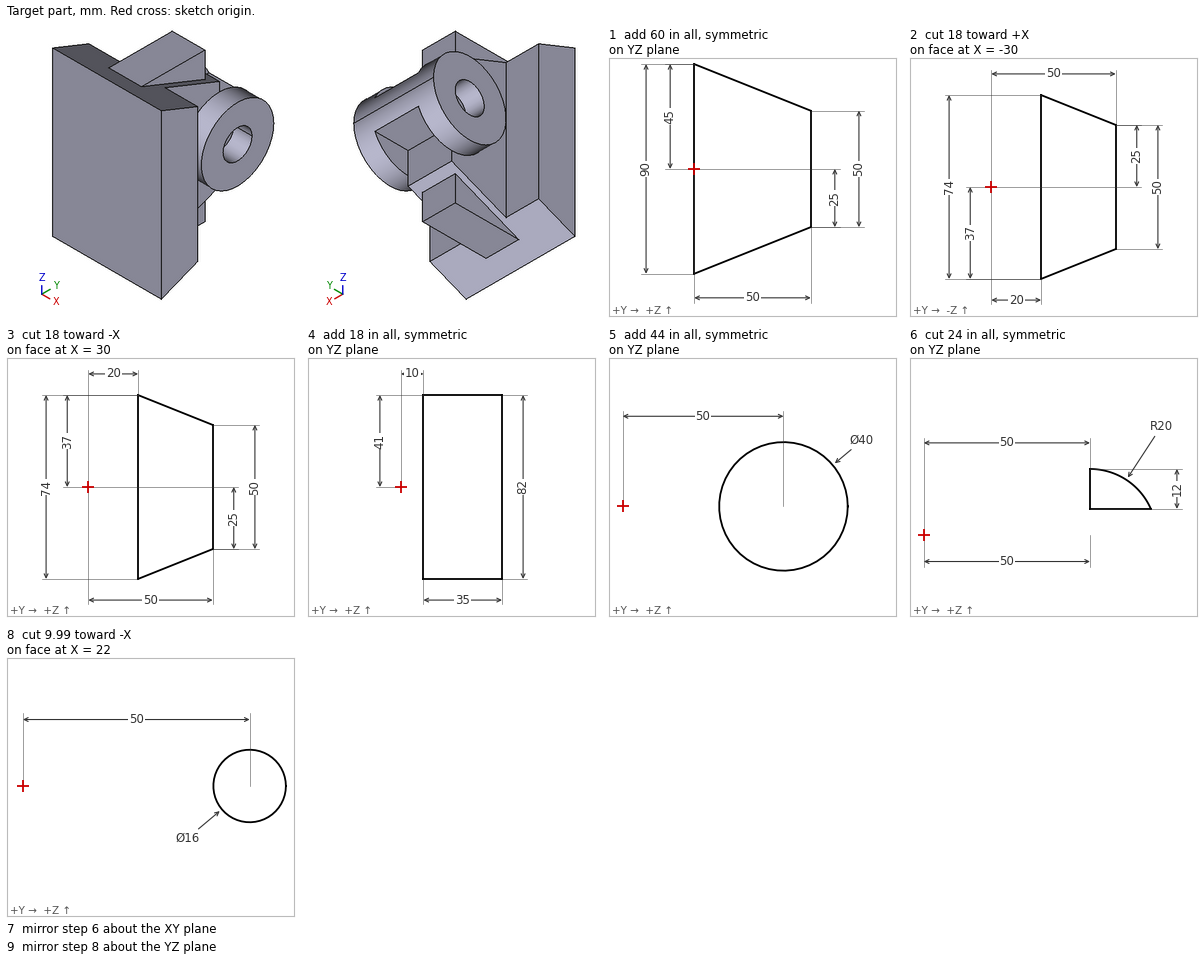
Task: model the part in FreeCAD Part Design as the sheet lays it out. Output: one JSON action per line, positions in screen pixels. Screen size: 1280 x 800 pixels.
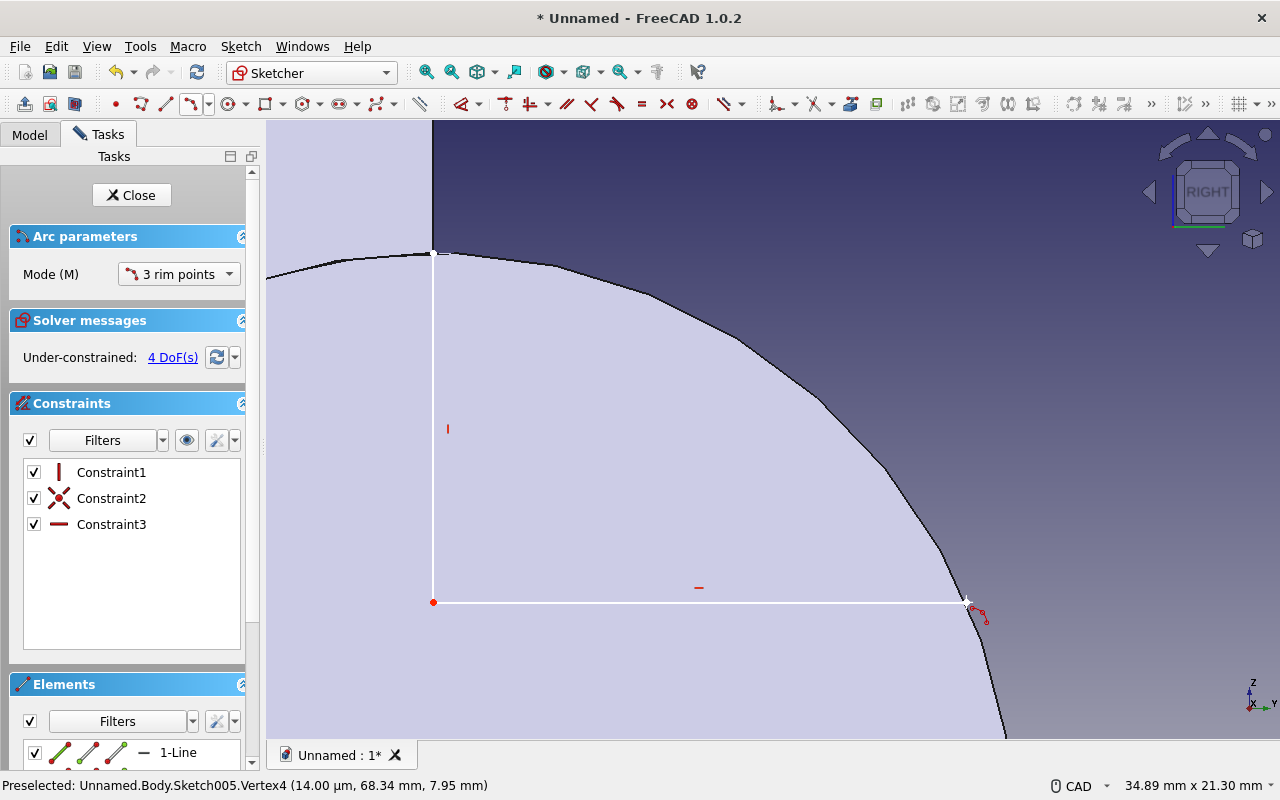
{"action": "left_click", "coordinate": [966, 603]}
{"action": "left_click", "coordinate": [433, 254]}
{"action": "left_click", "coordinate": [751, 348]}
{"action": "key", "text": "Escape"}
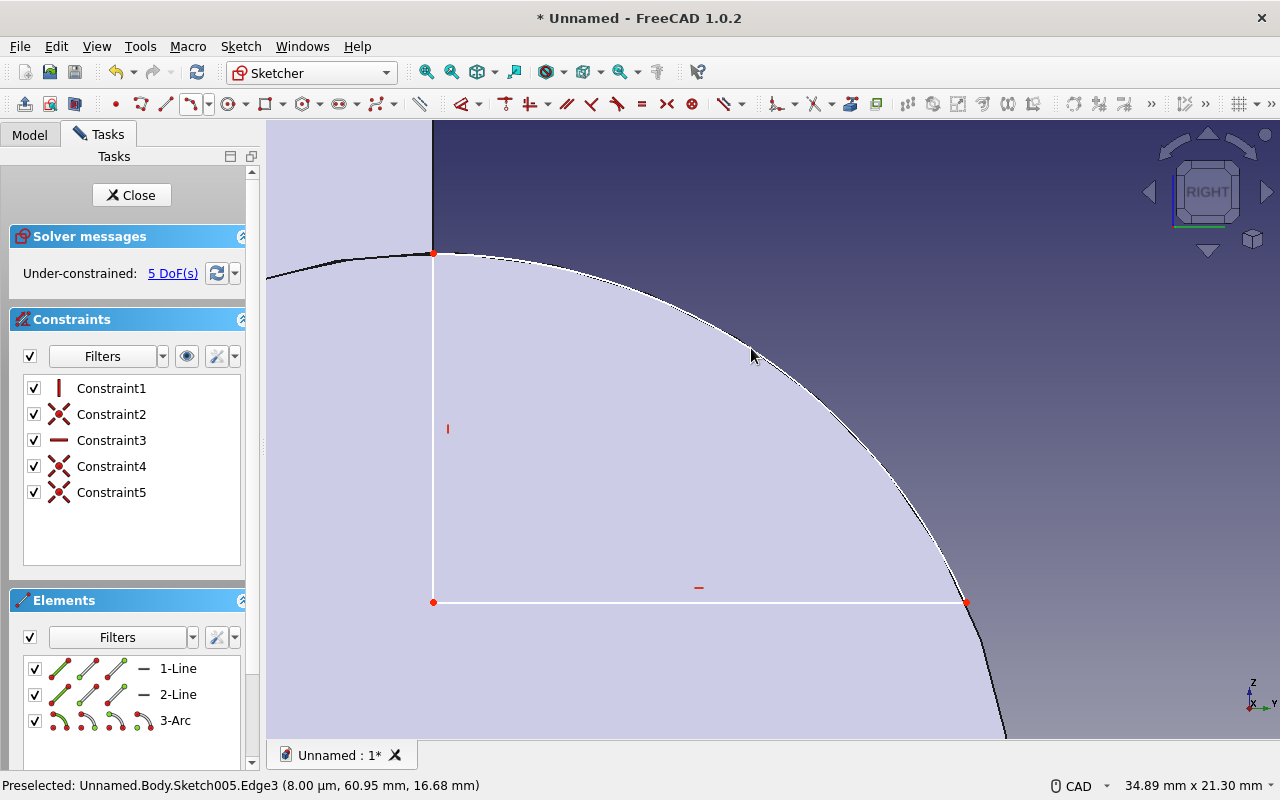
{"action": "scroll", "coordinate": [716, 195], "scroll_direction": "down", "scroll_amount": 2}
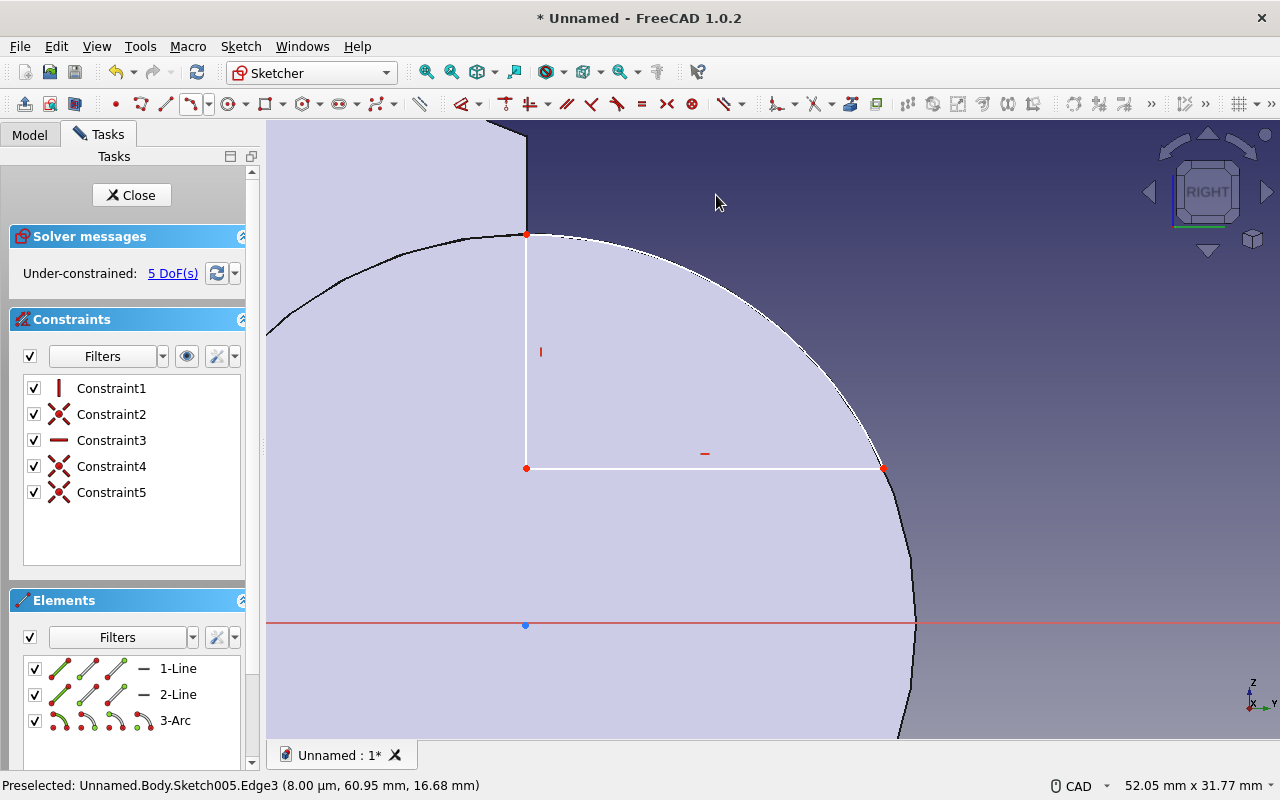
{"action": "left_click", "coordinate": [526, 625]}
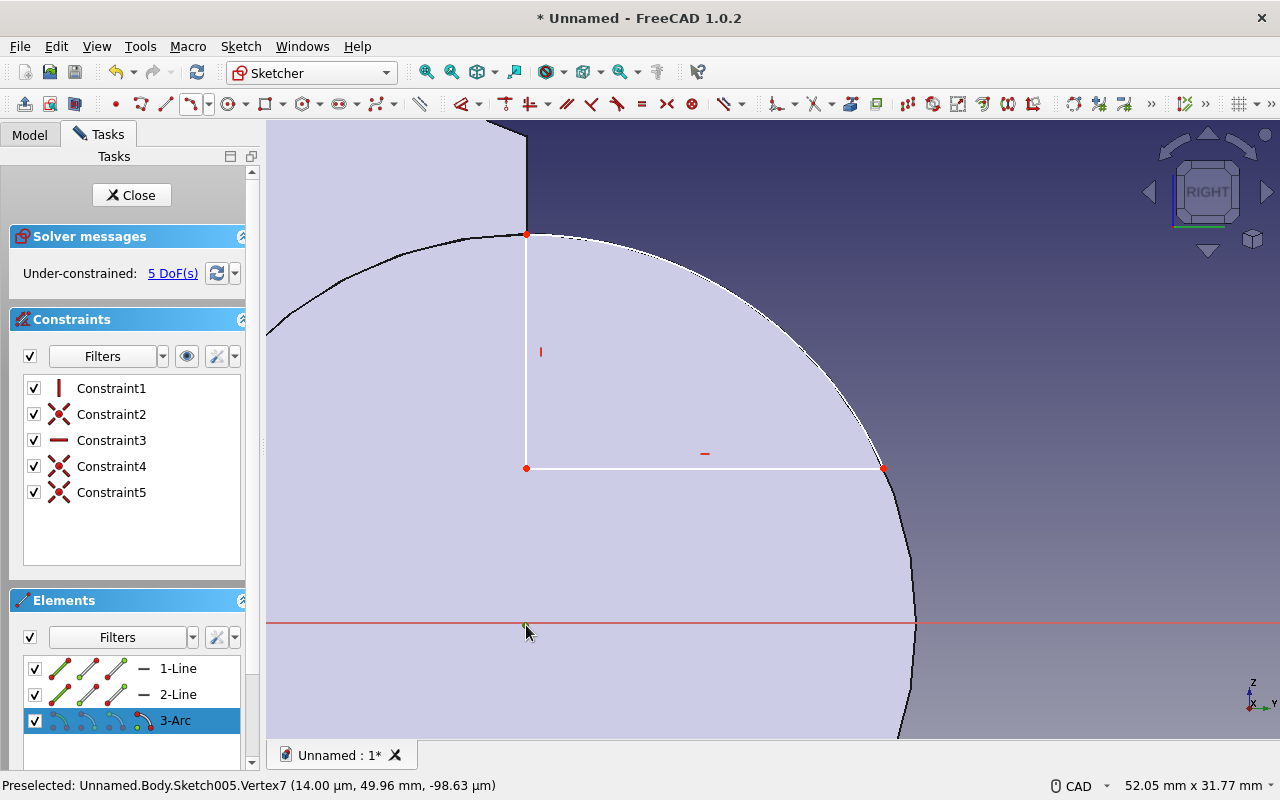
{"action": "left_click", "coordinate": [353, 623]}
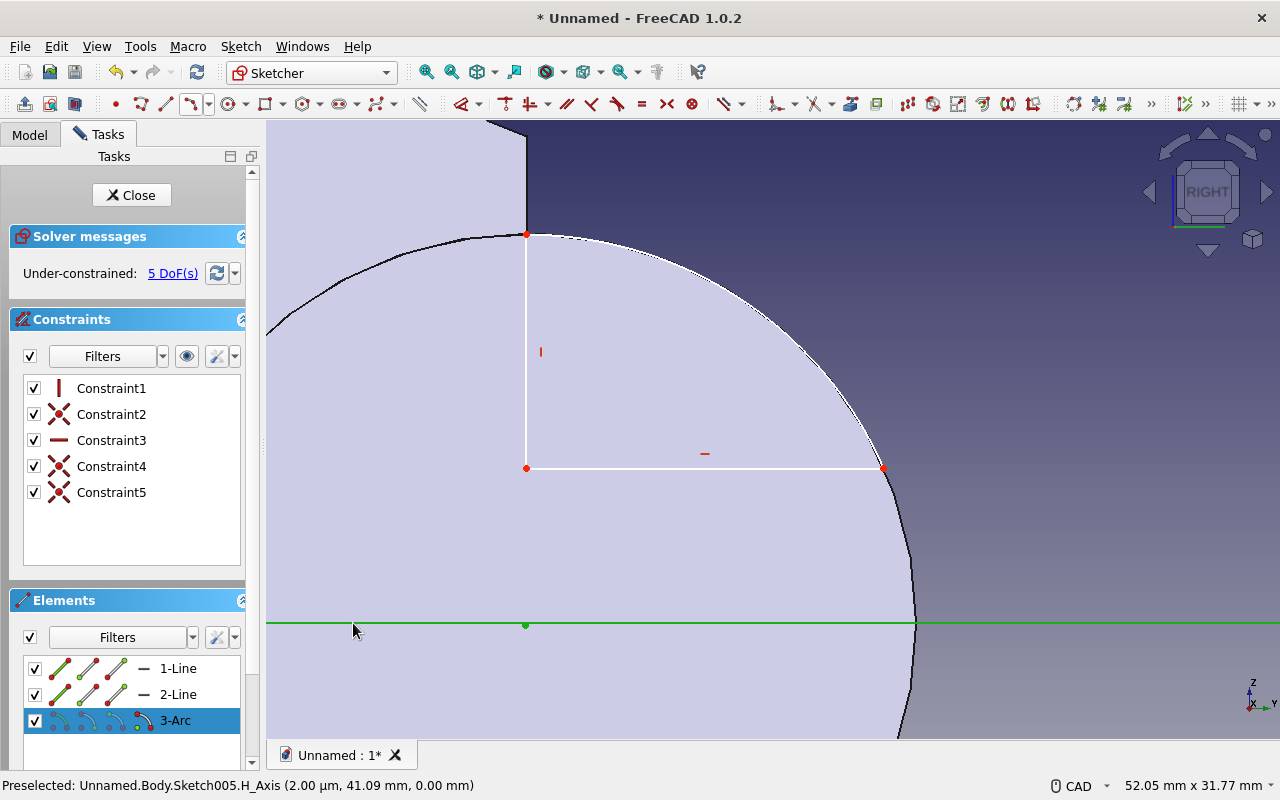
{"action": "left_click", "coordinate": [505, 104]}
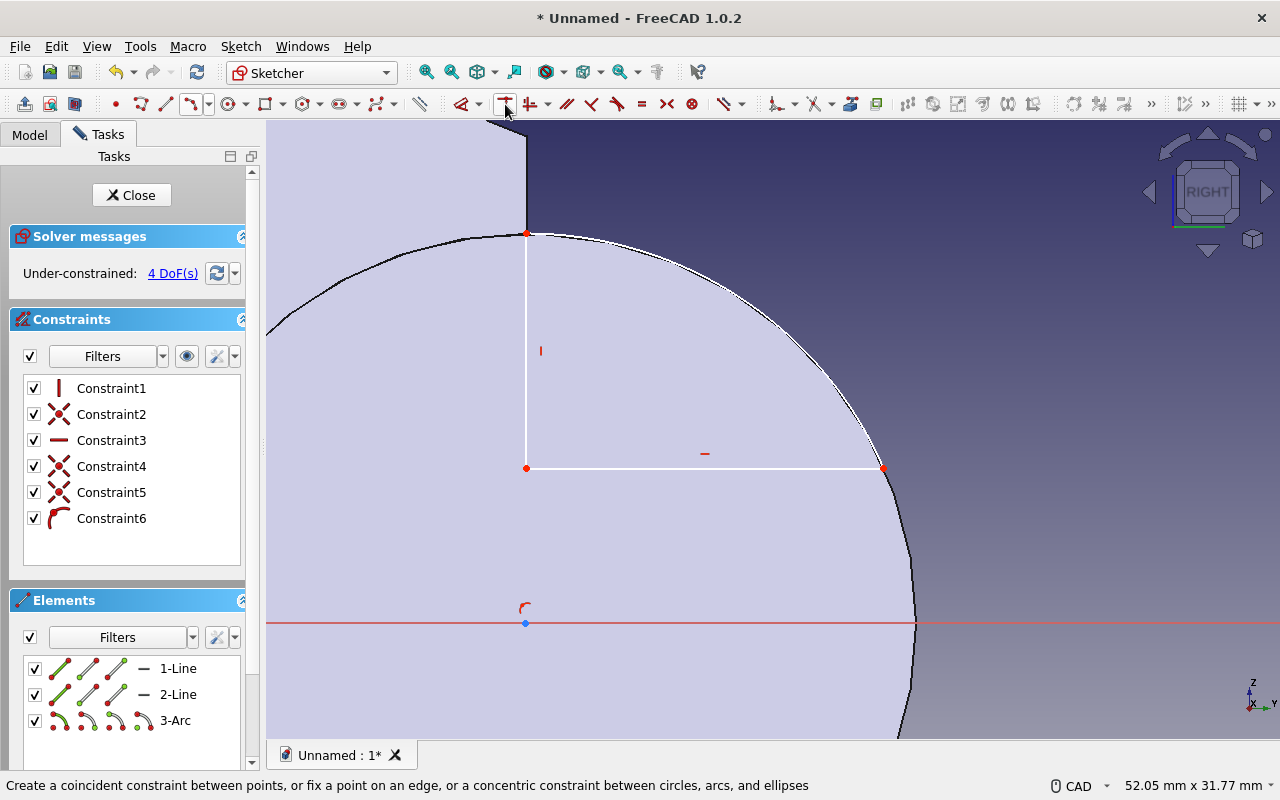
{"action": "left_click", "coordinate": [460, 104]}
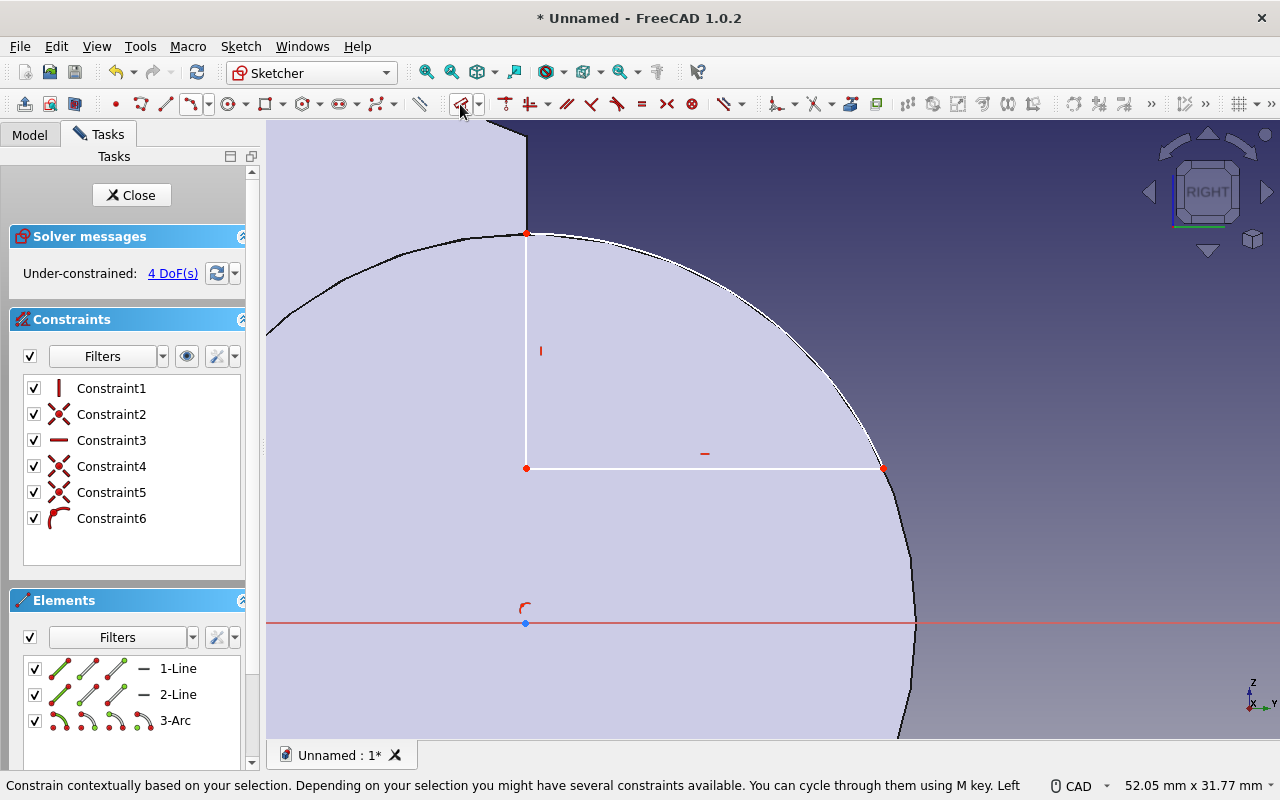
{"action": "left_click", "coordinate": [809, 356]}
{"action": "left_click", "coordinate": [832, 334]}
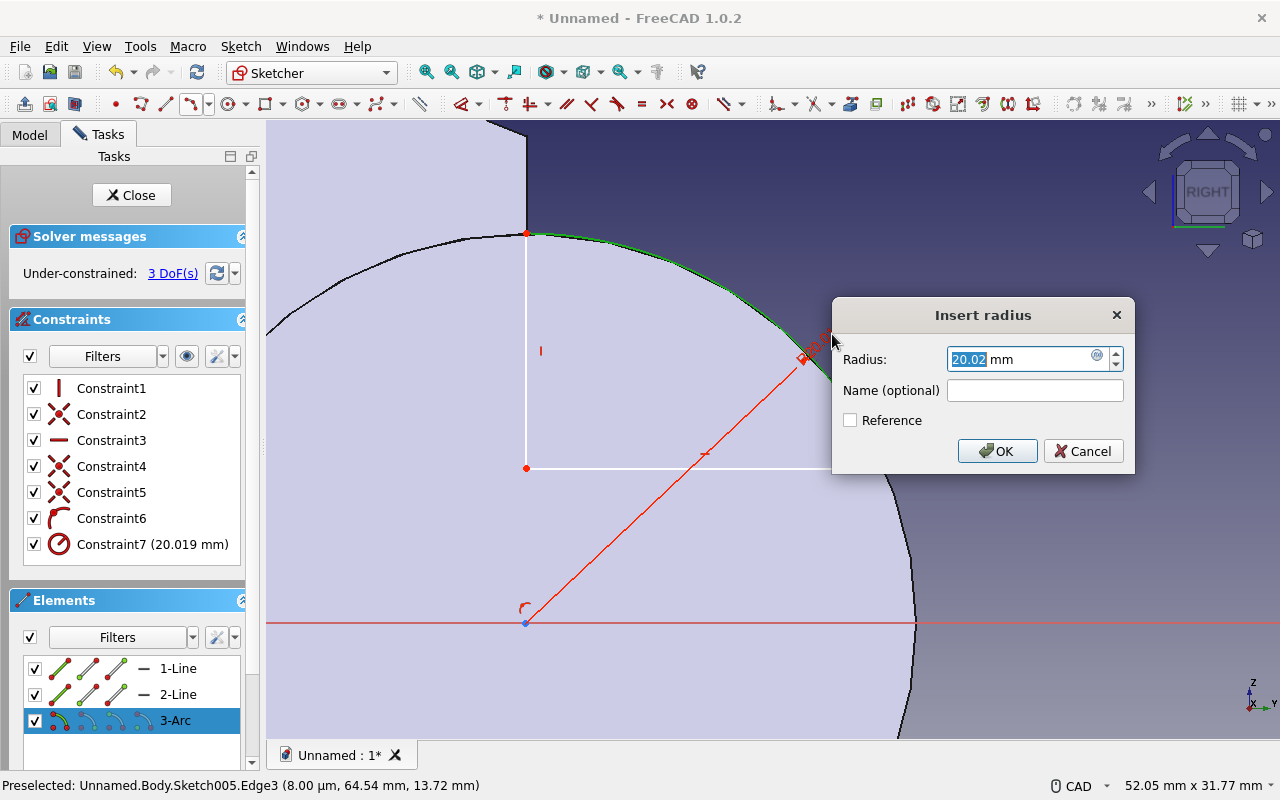
{"action": "type", "text": "20"}
{"action": "key", "text": "Return"}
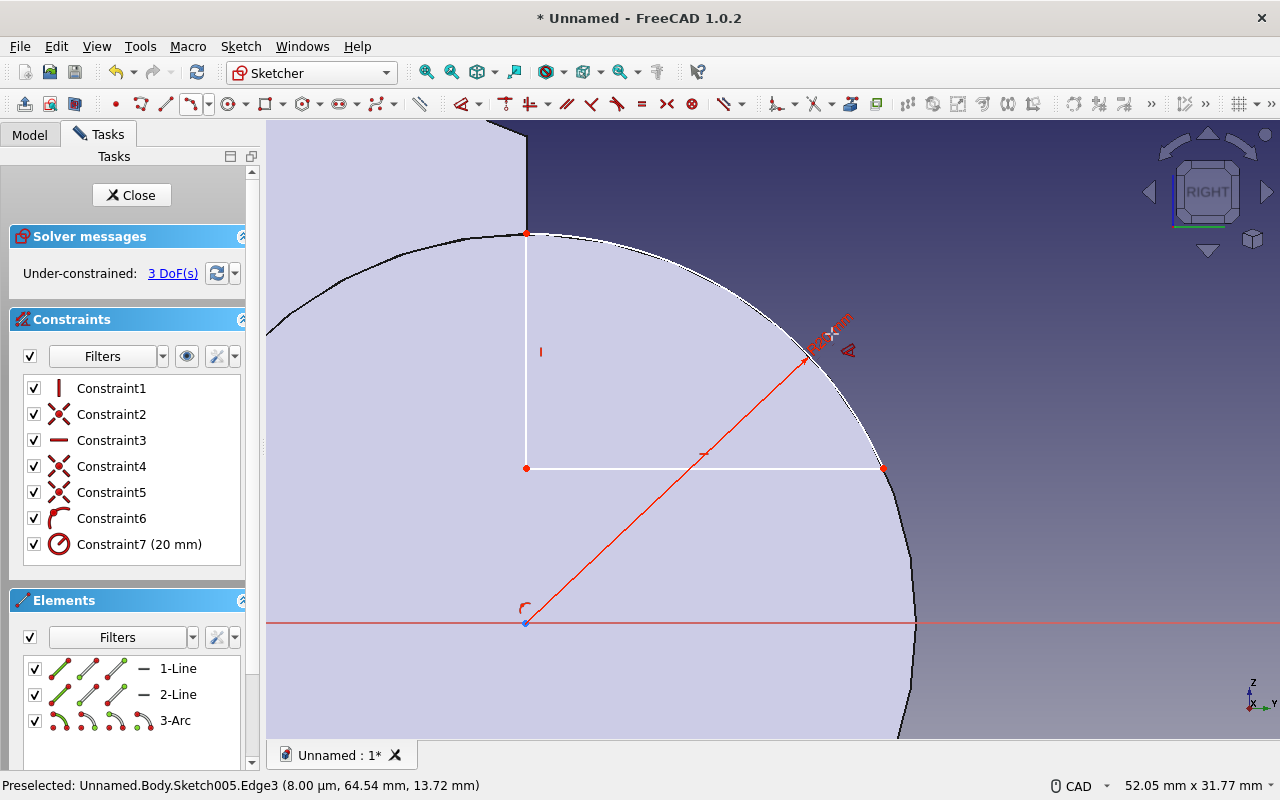
{"action": "left_click", "coordinate": [526, 304]}
{"action": "left_click", "coordinate": [492, 351]}